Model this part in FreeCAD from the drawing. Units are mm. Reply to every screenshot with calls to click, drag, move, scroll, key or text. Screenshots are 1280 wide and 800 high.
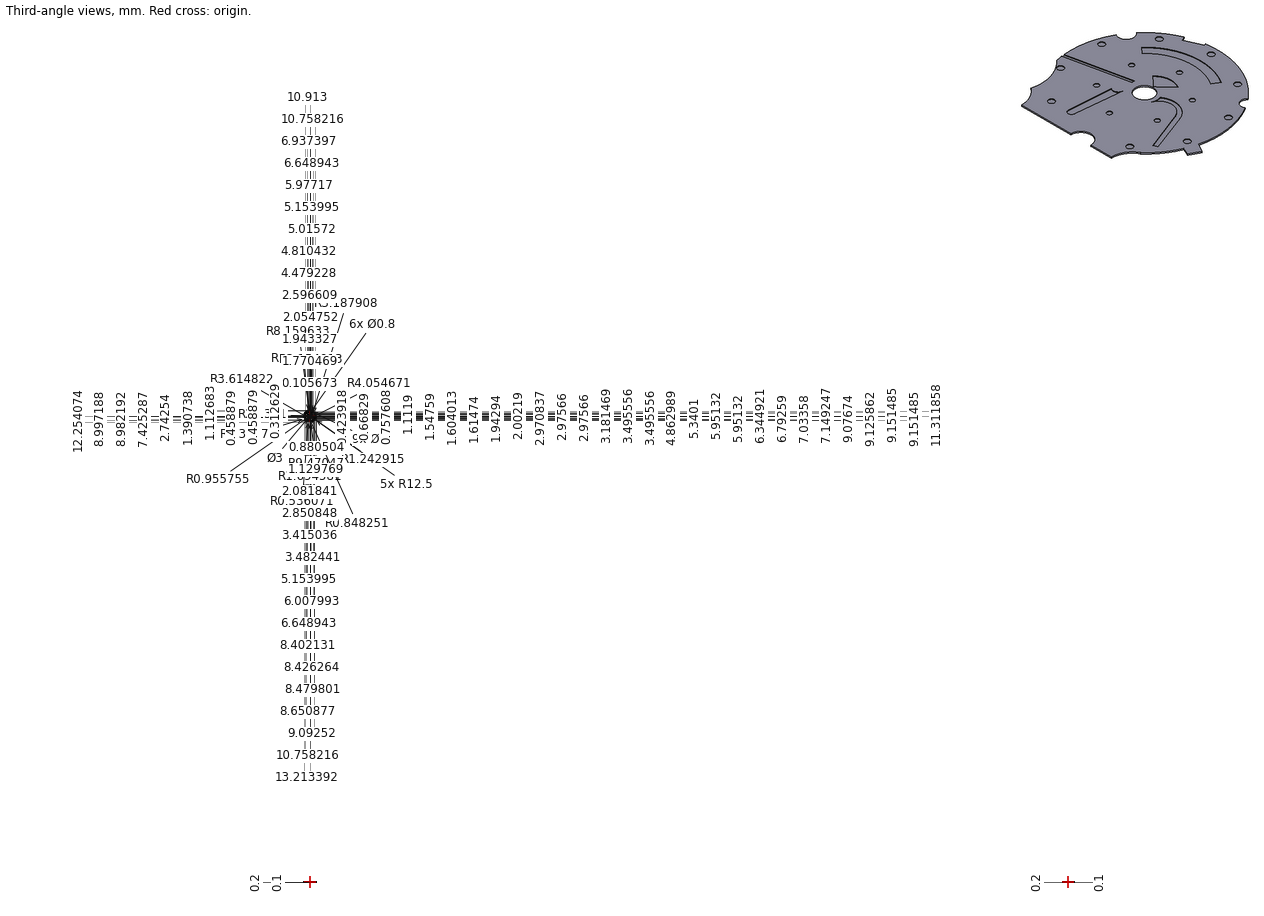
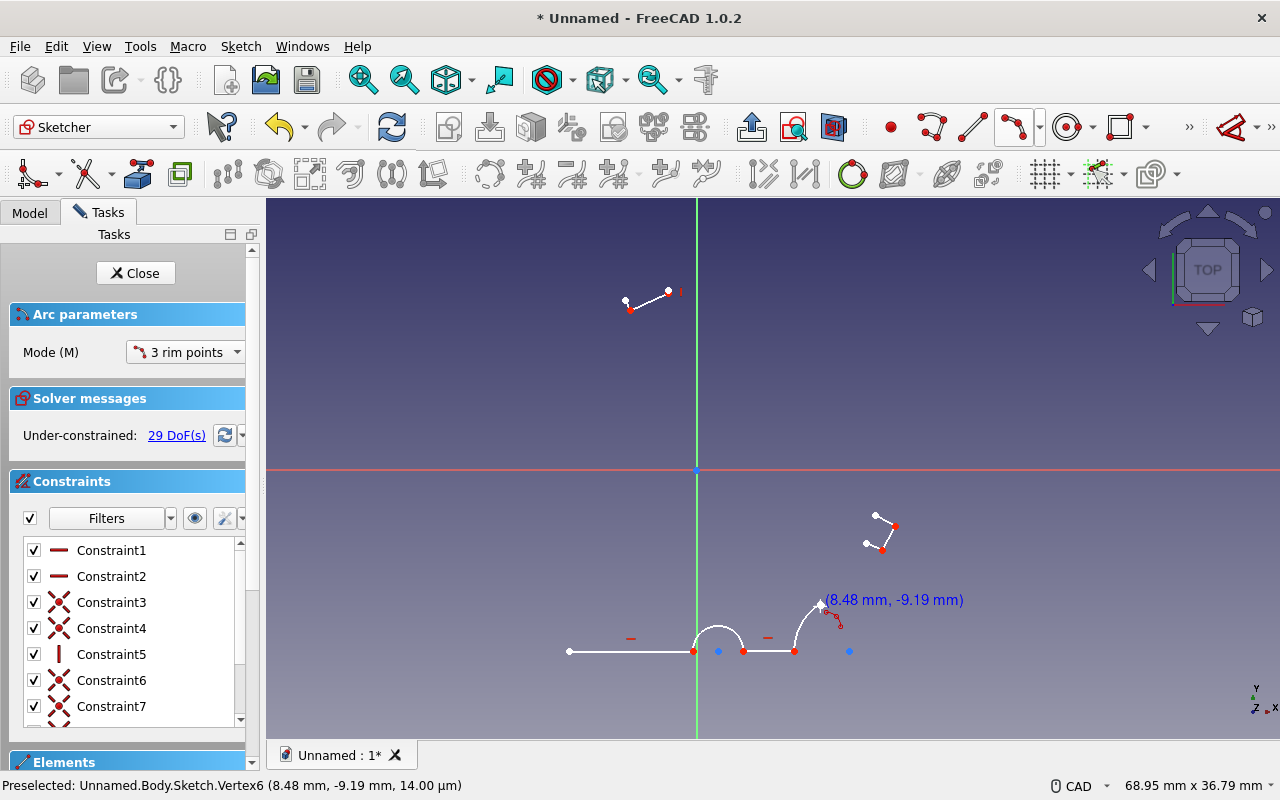
scroll(866, 542, up, 3)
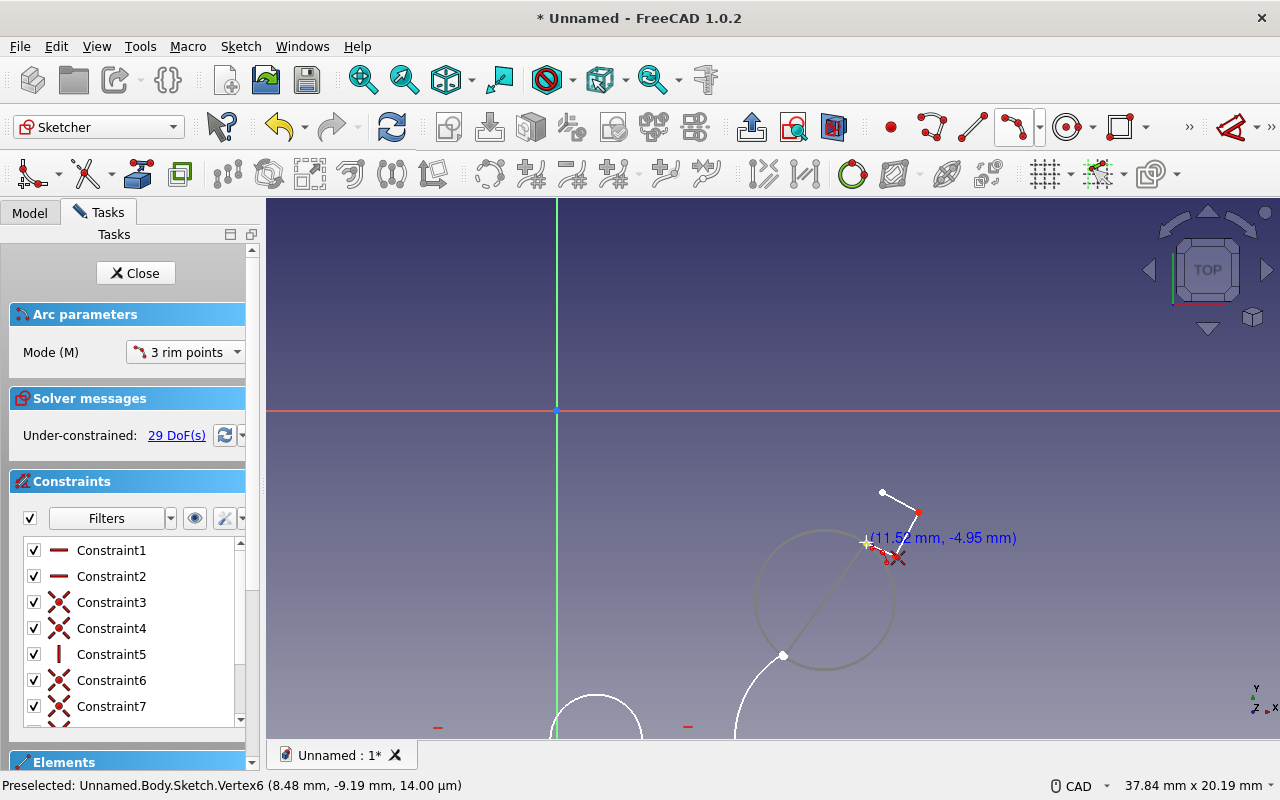
click(866, 543)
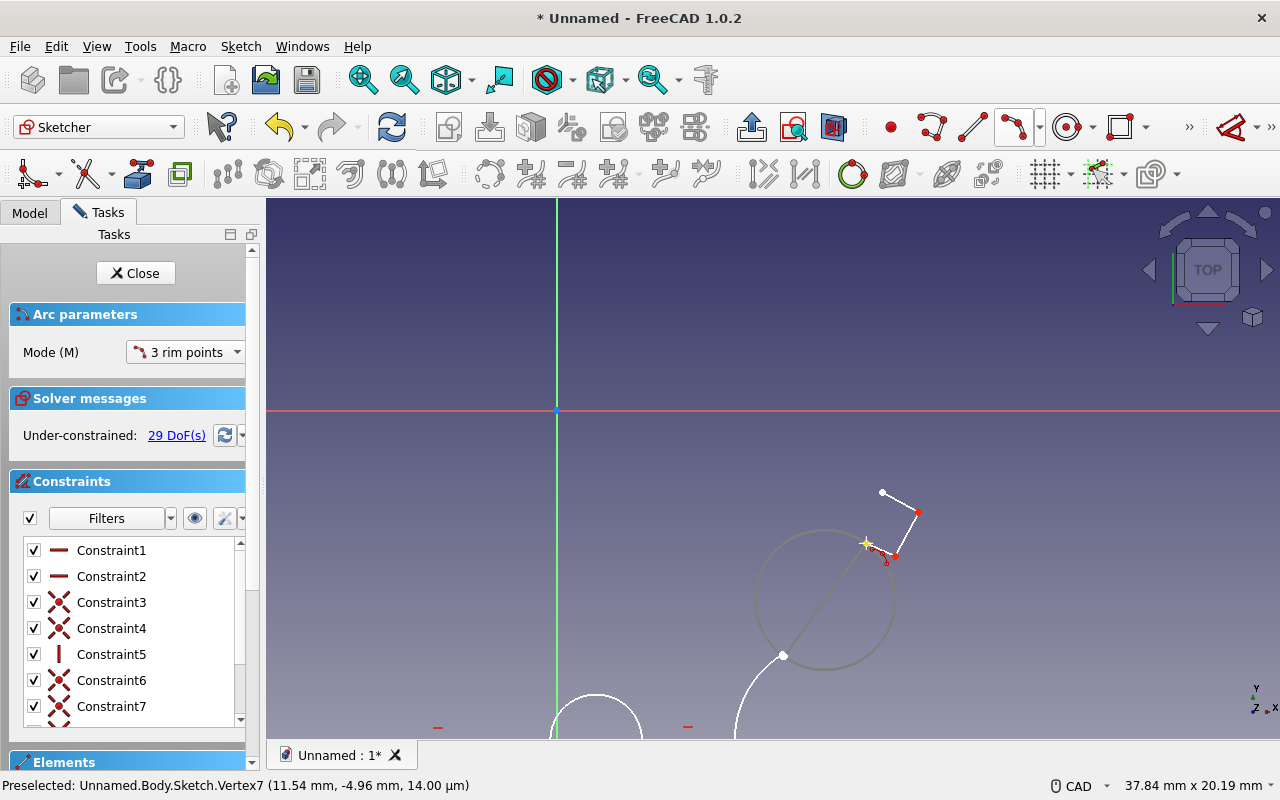
scroll(831, 603, up, 4)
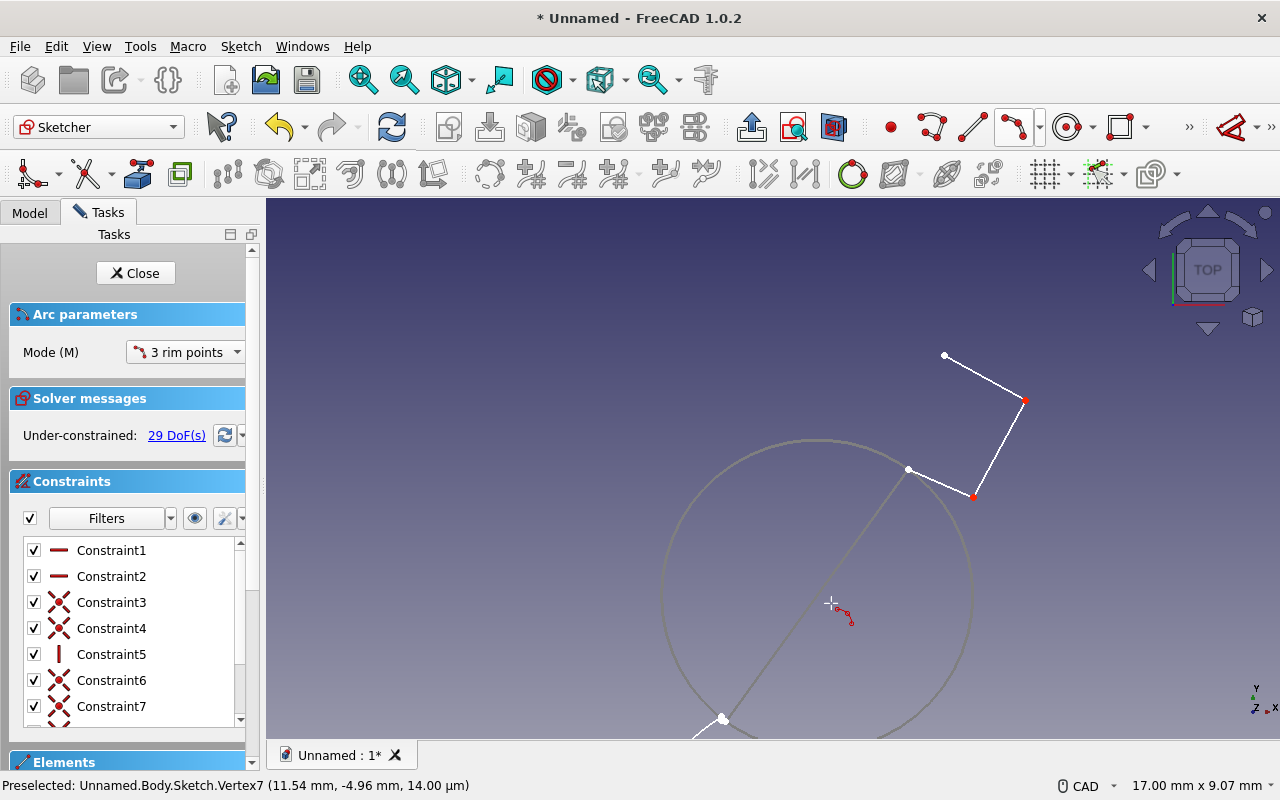
click(830, 602)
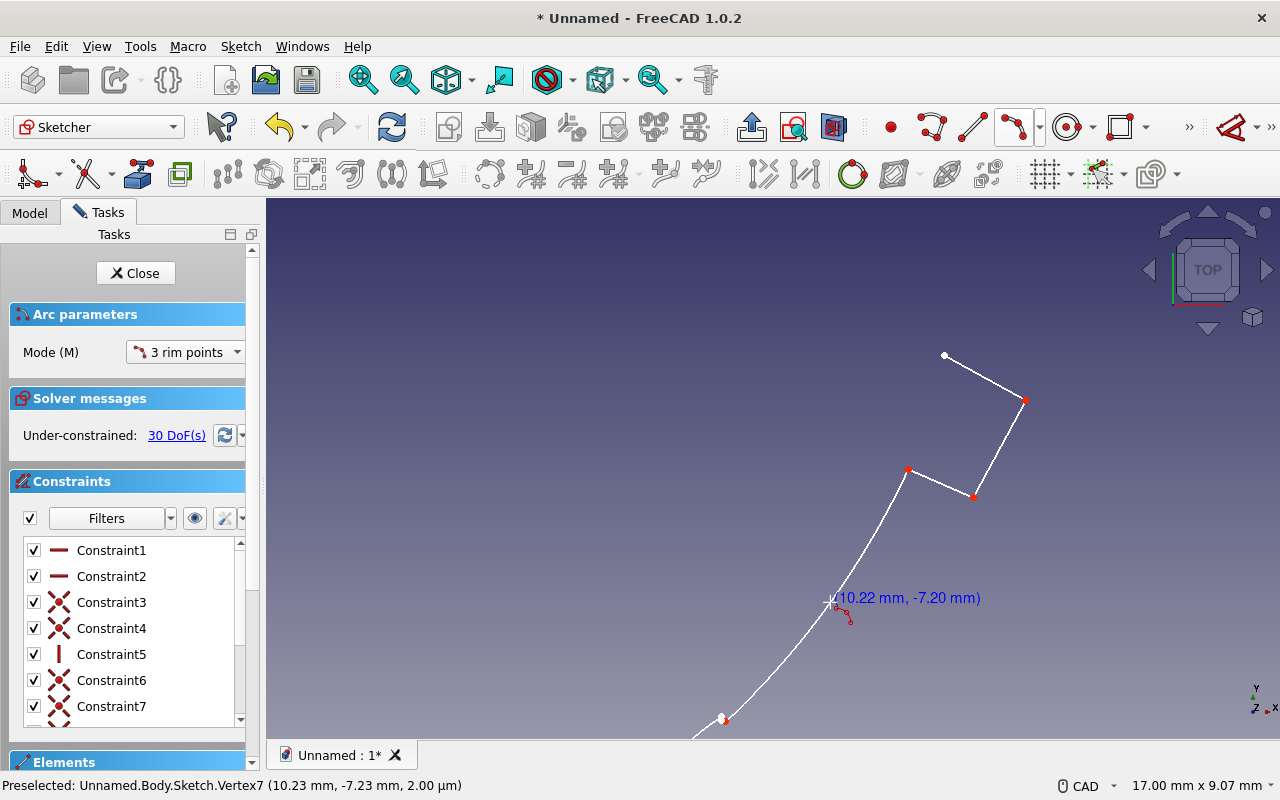
scroll(852, 566, down, 7)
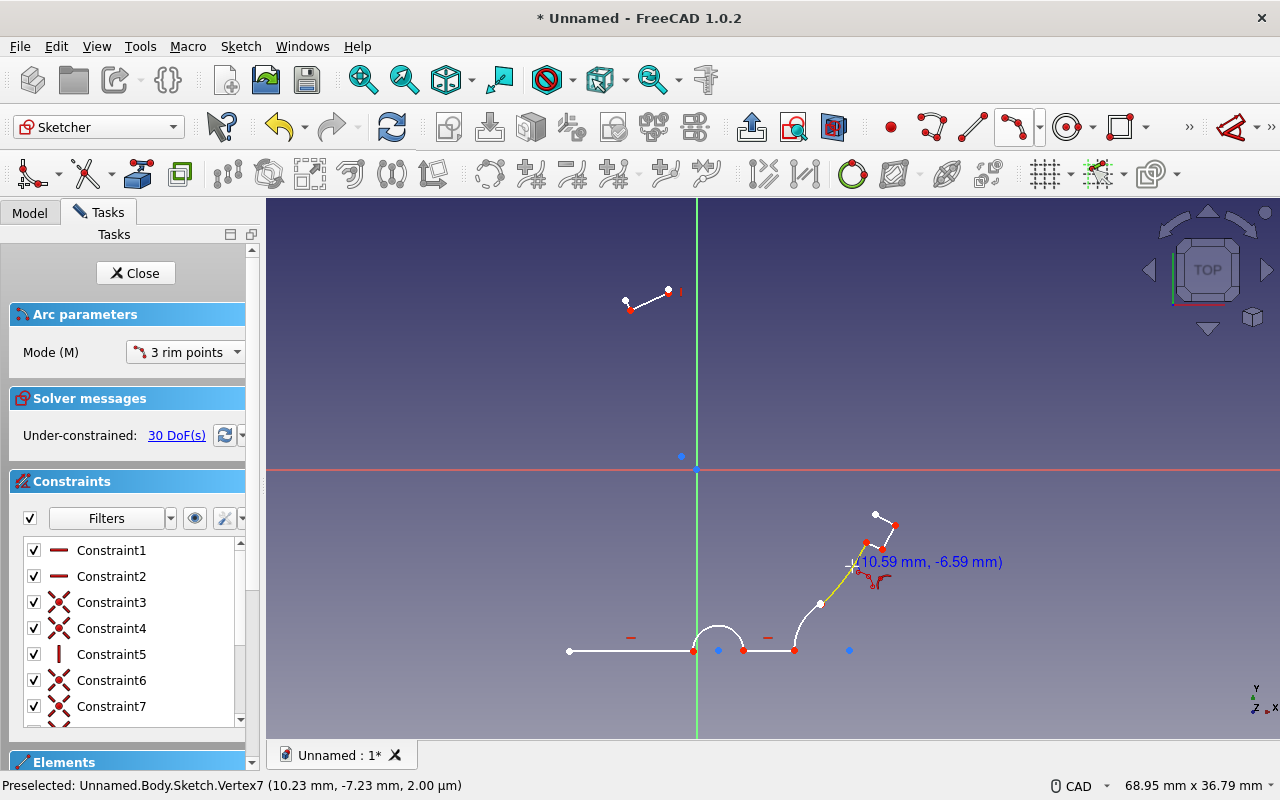
scroll(875, 513, up, 2)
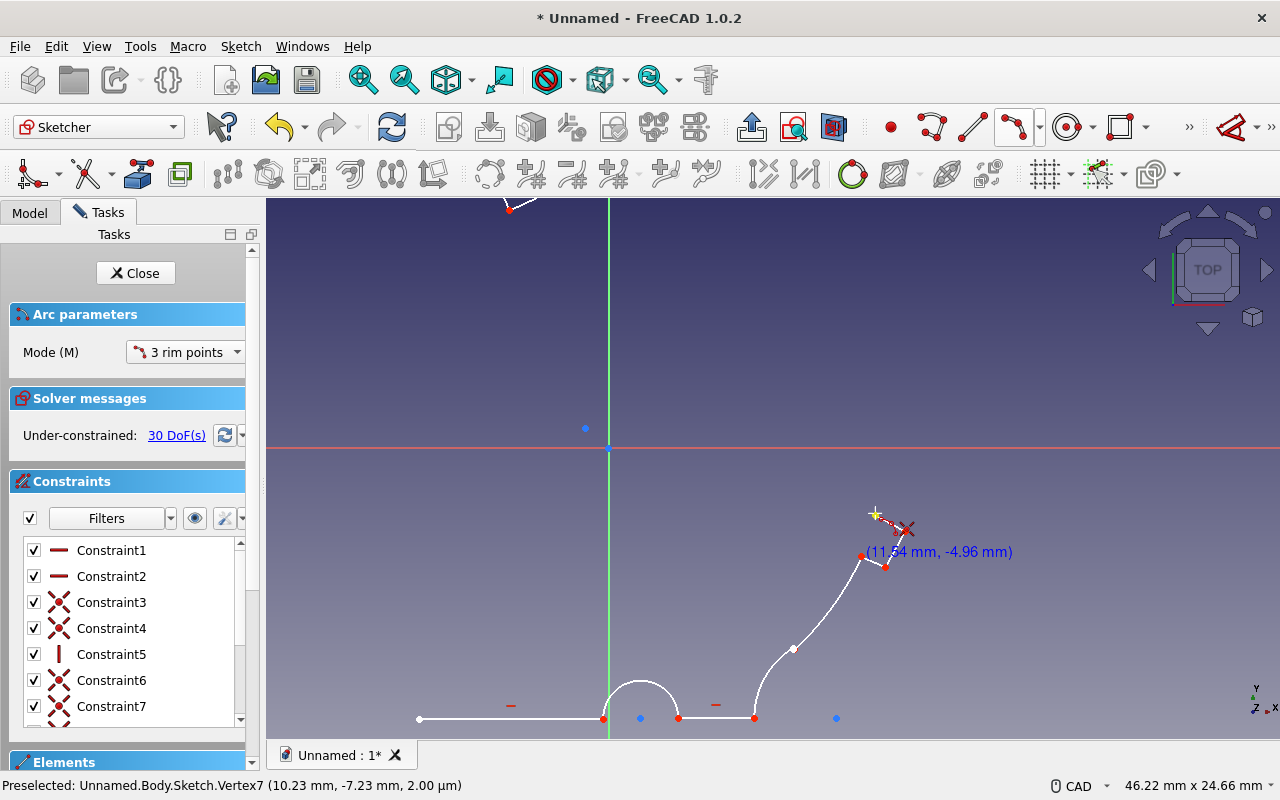
click(875, 515)
click(845, 309)
click(880, 408)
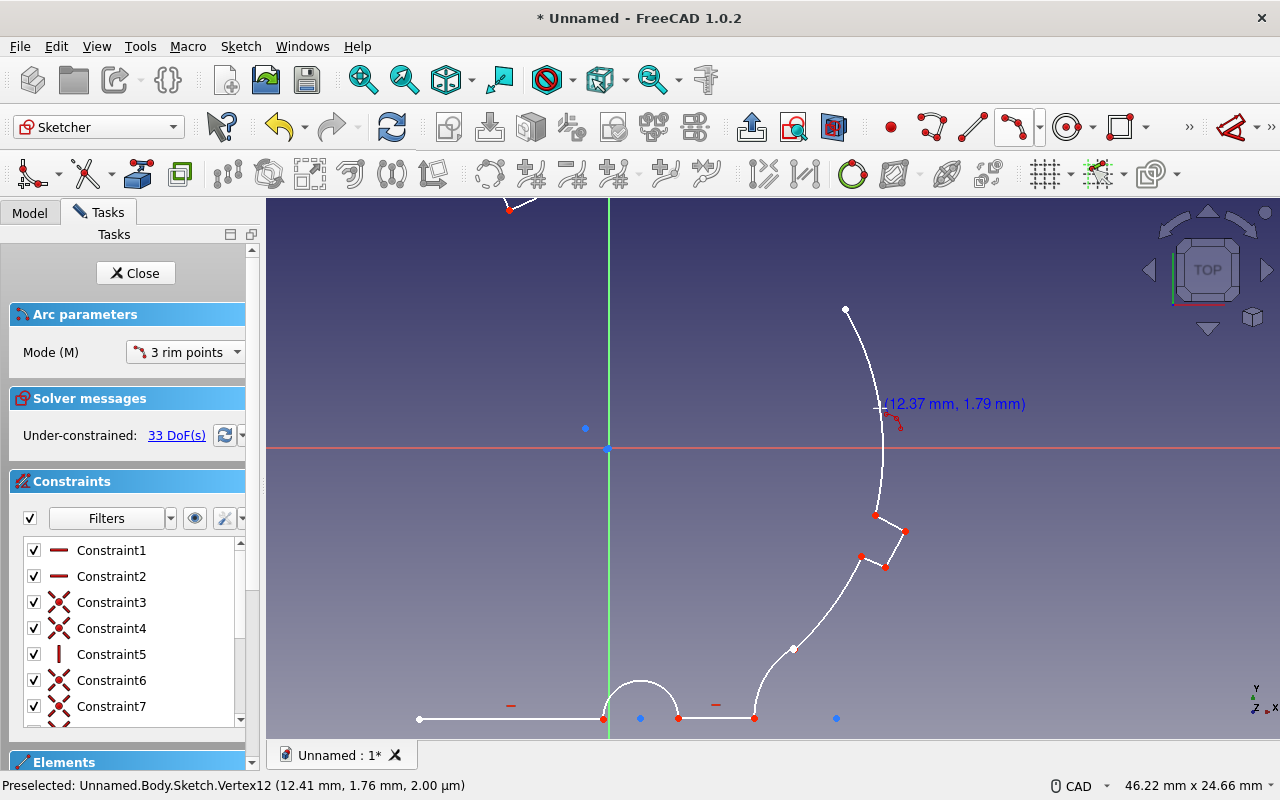
click(845, 310)
click(821, 275)
click(816, 303)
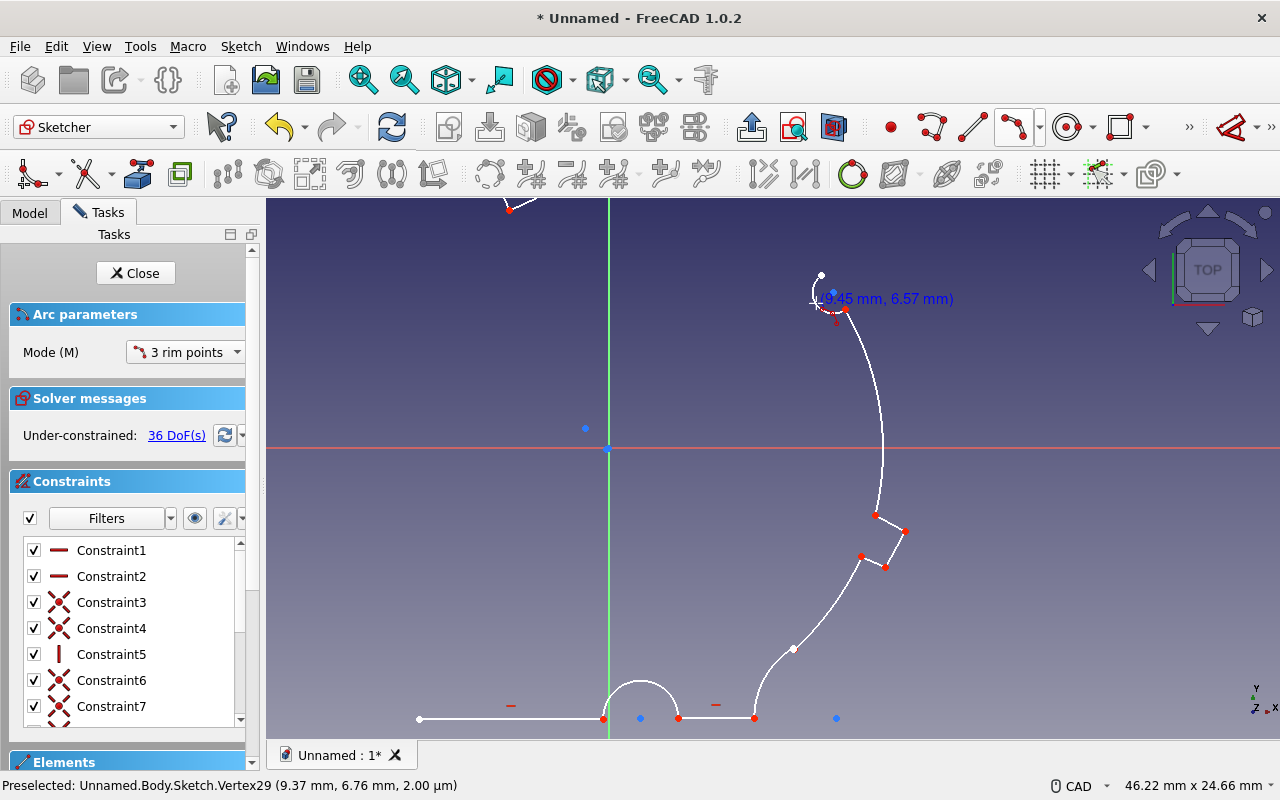
click(821, 276)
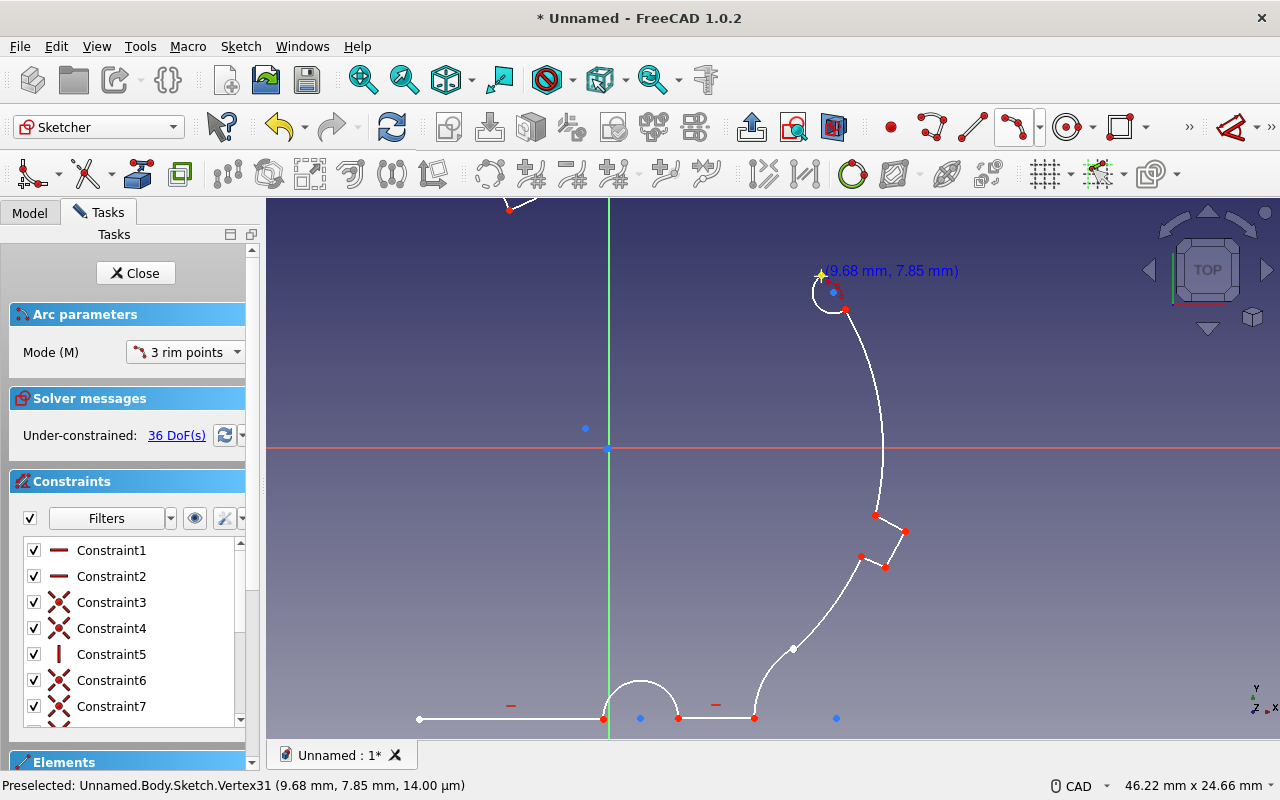
scroll(874, 512, down, 2)